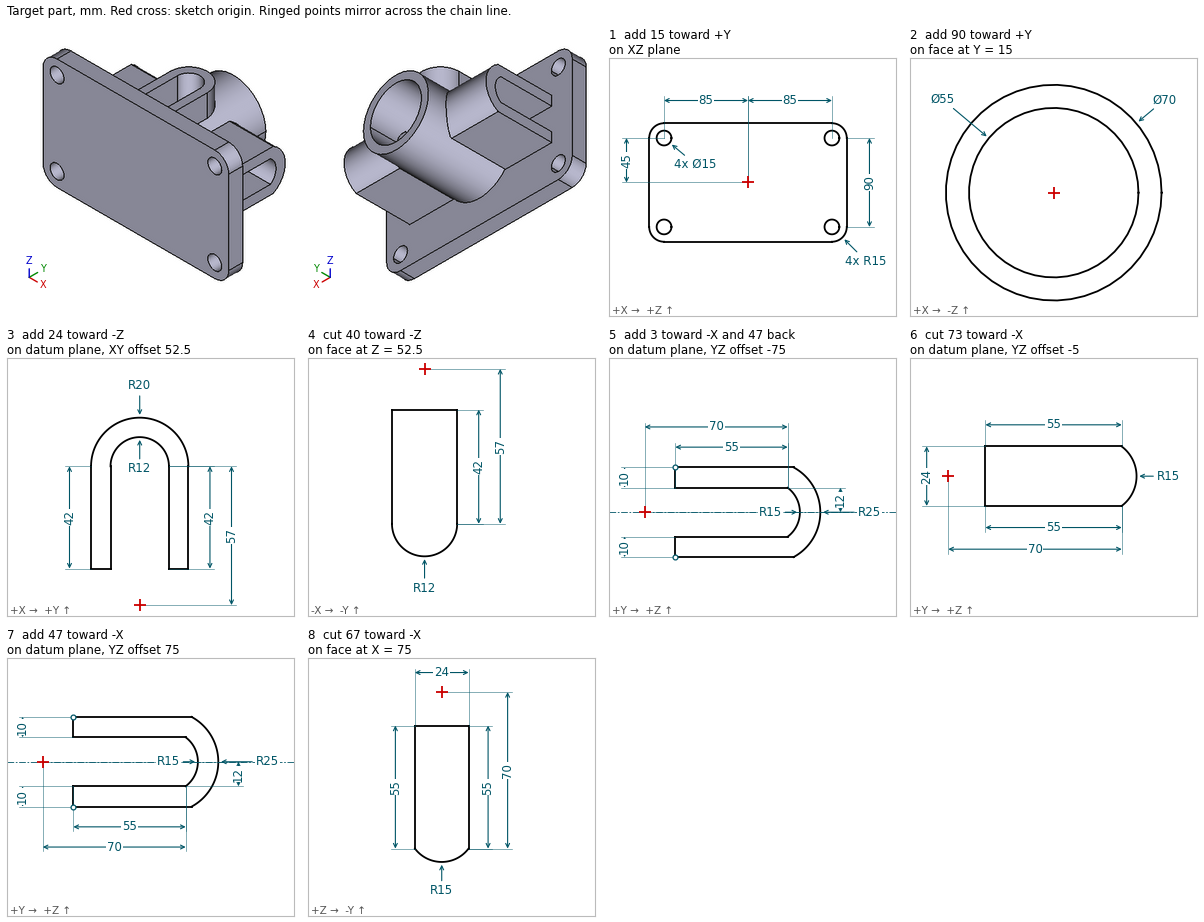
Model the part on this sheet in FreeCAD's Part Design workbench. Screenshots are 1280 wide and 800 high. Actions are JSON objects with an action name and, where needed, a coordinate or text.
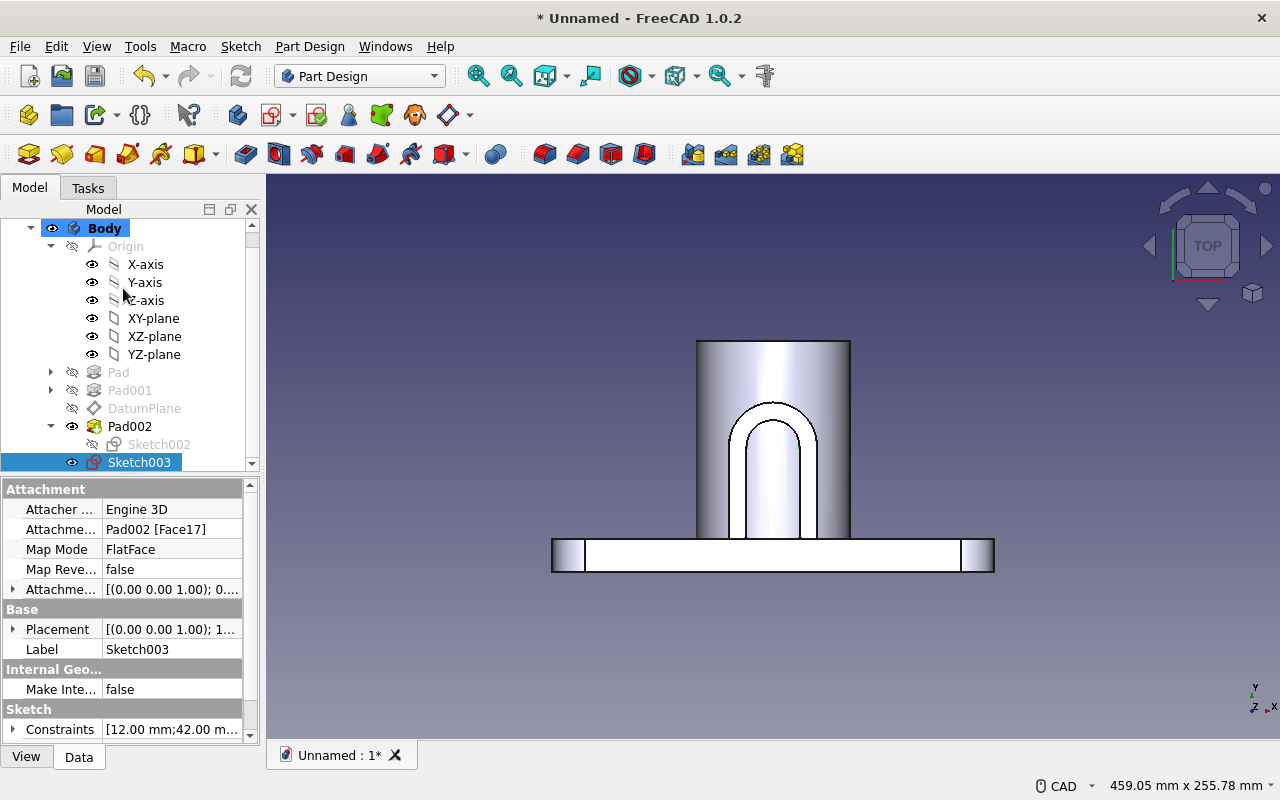
{"action": "left_click", "coordinate": [246, 154]}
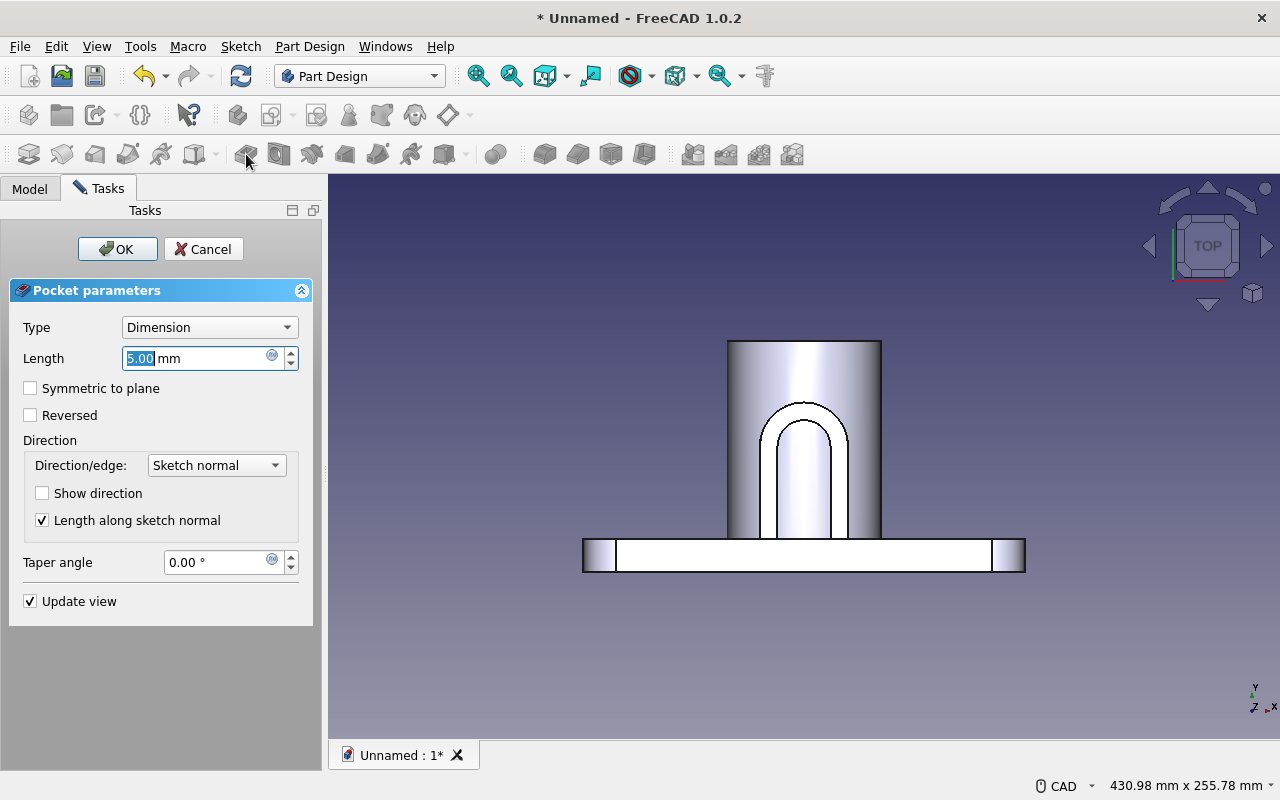
{"action": "type", "text": "40"}
{"action": "key", "text": "Tab"}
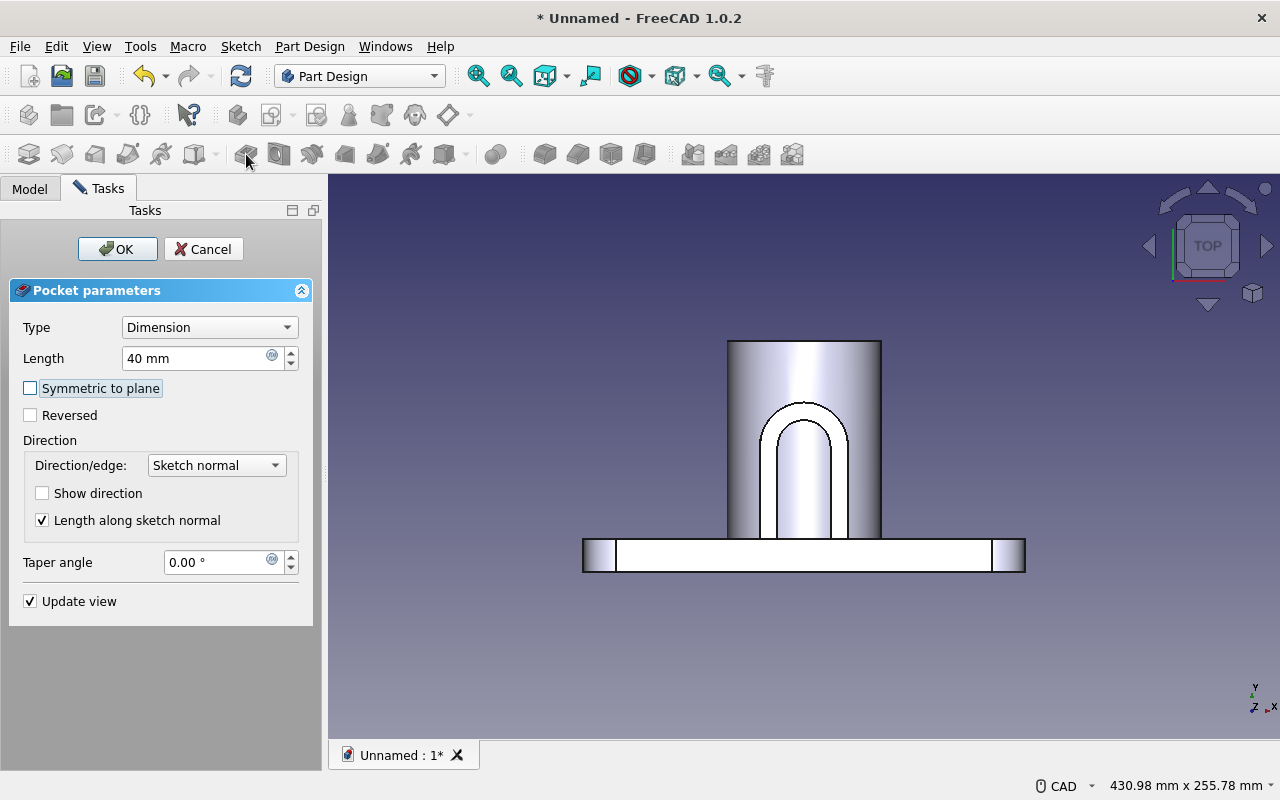
{"action": "left_click", "coordinate": [118, 249]}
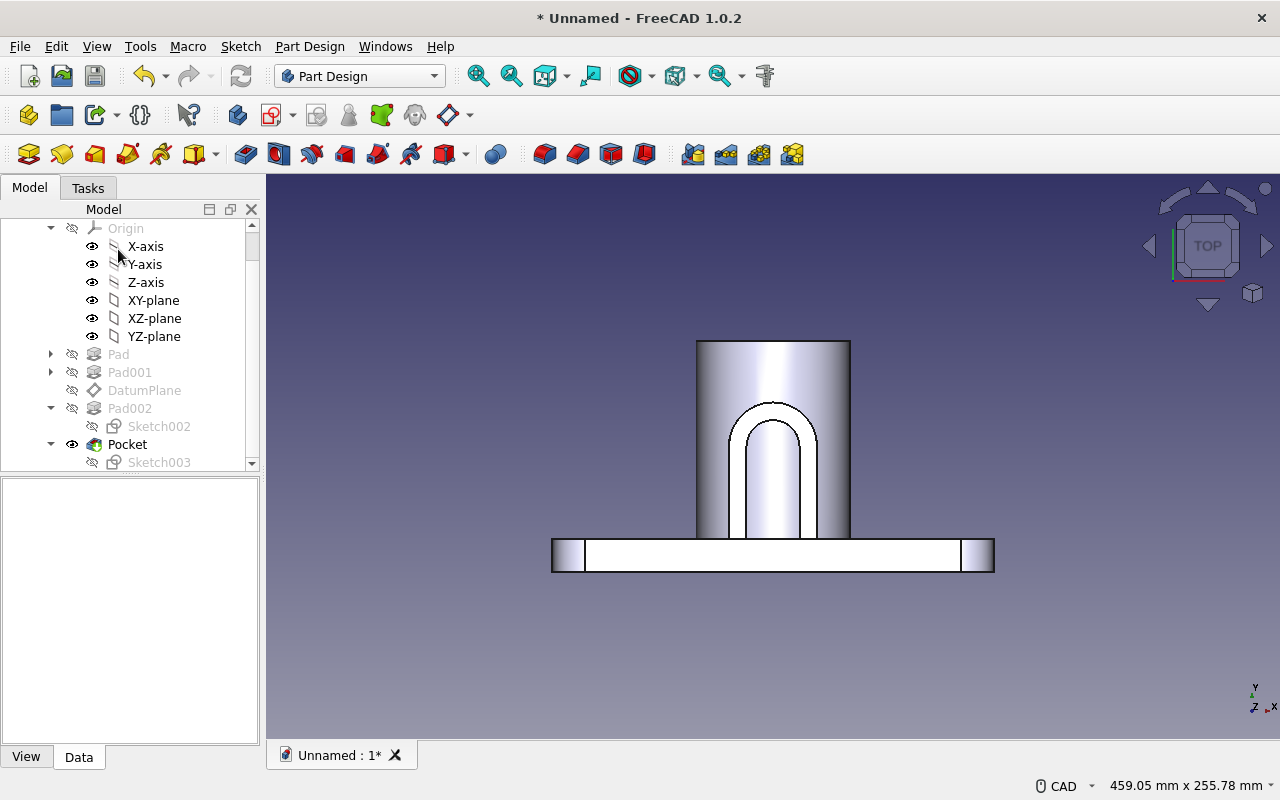
{"action": "left_click", "coordinate": [479, 76]}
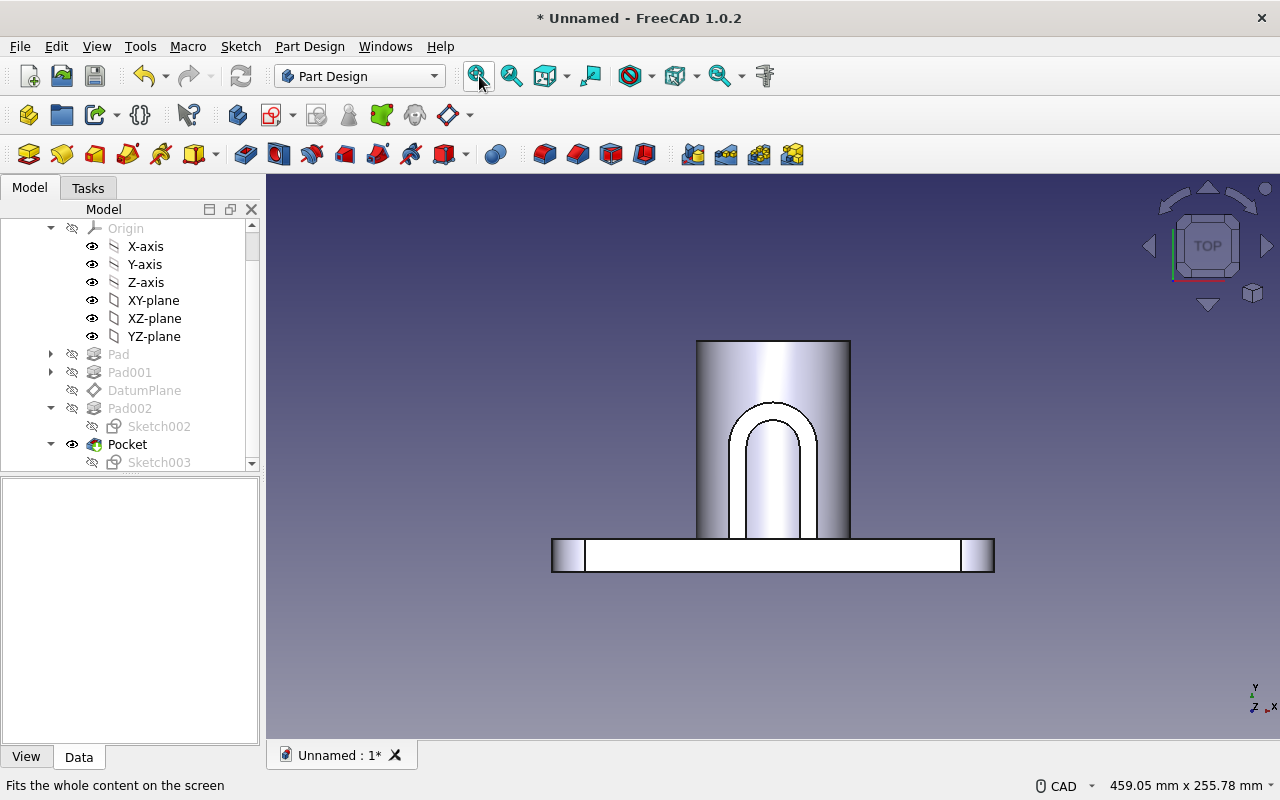
{"action": "left_click", "coordinate": [137, 336]}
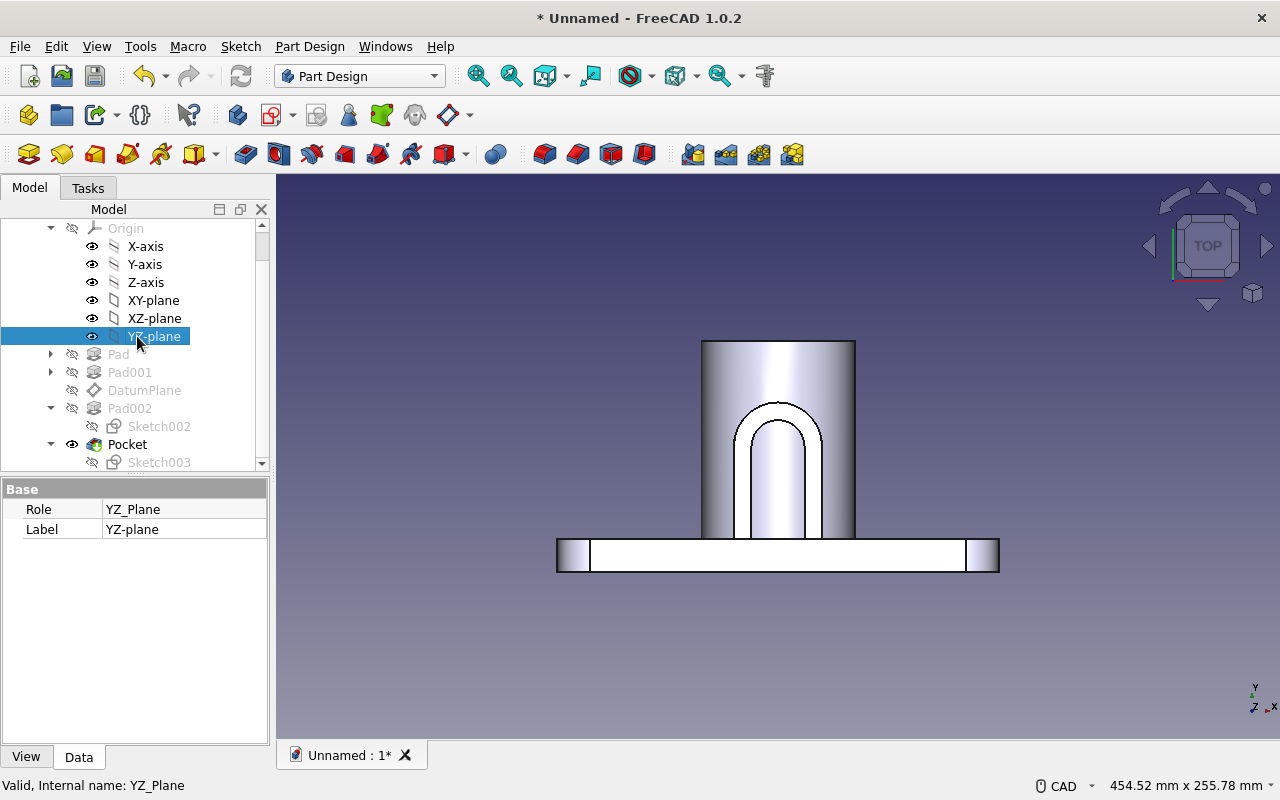
{"action": "left_click", "coordinate": [448, 116]}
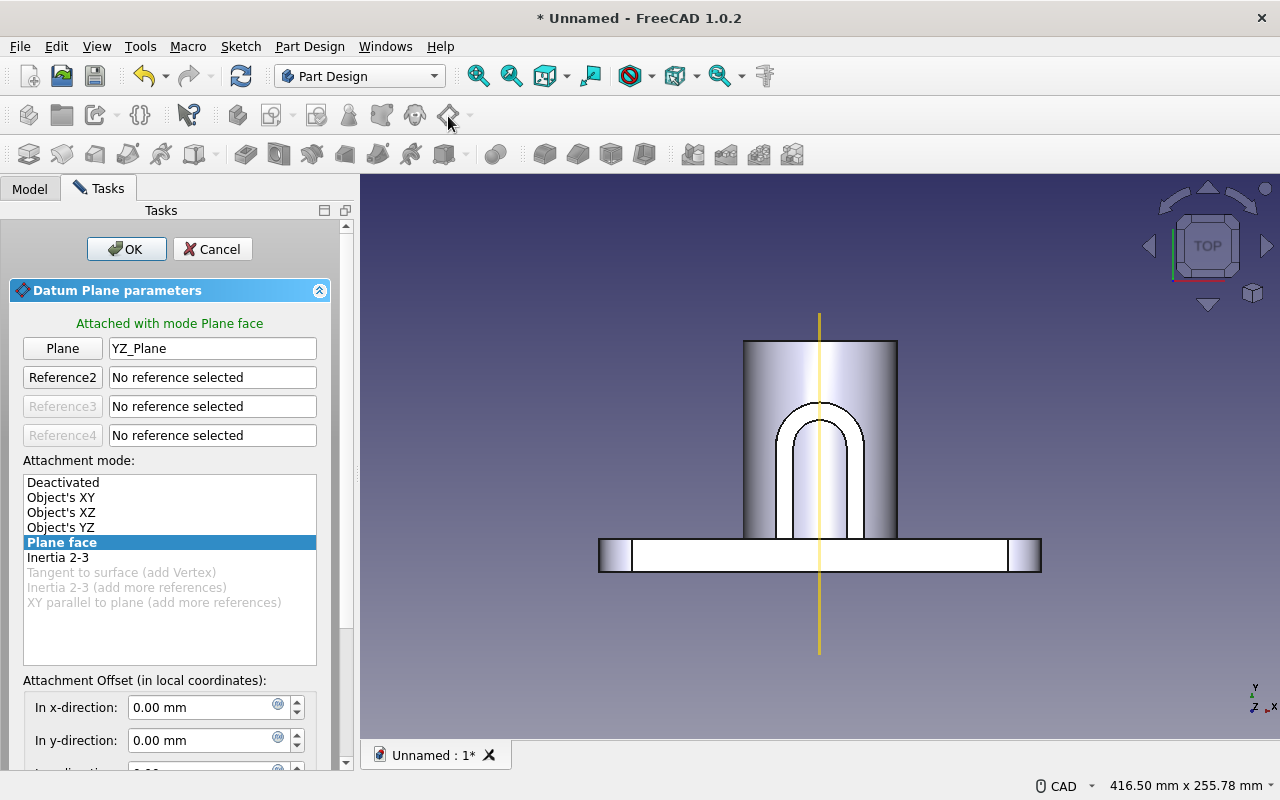
{"action": "scroll", "coordinate": [346, 495], "scroll_direction": "down", "scroll_amount": 2}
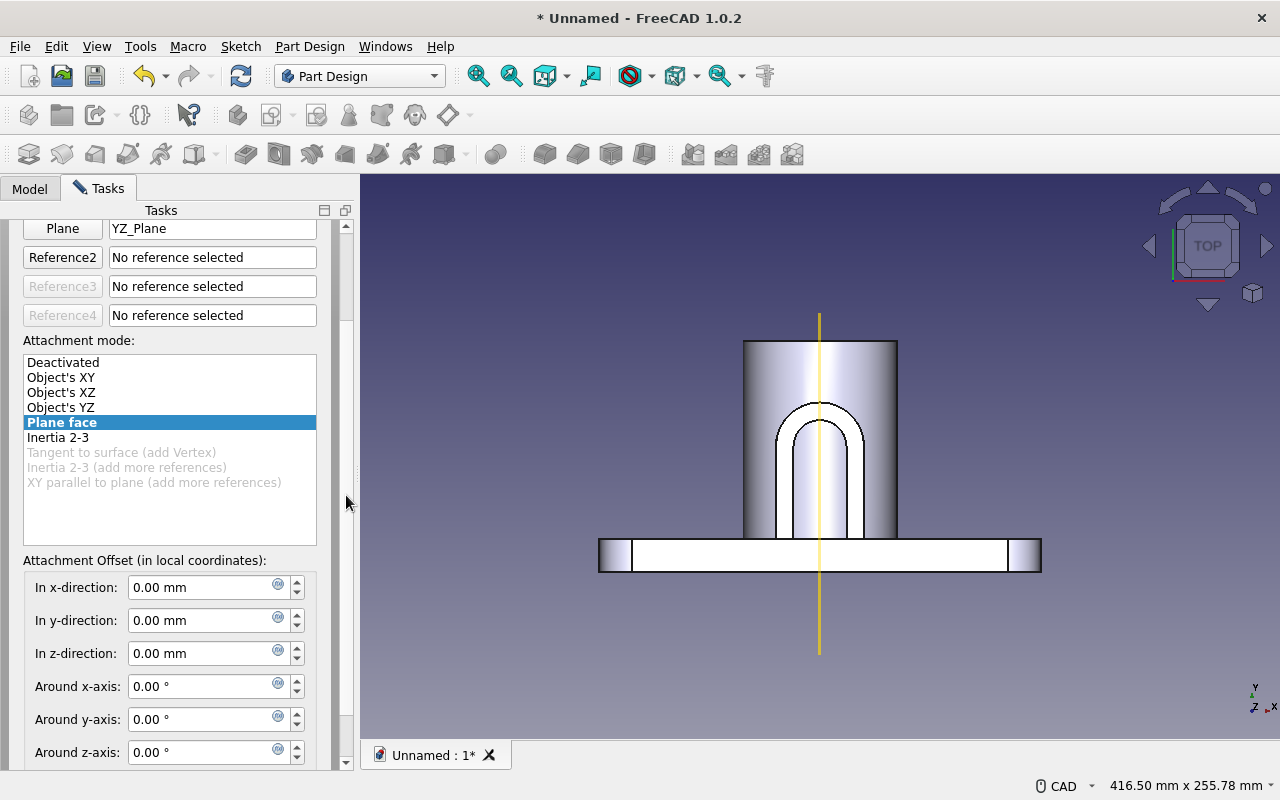
{"action": "triple_click", "coordinate": [210, 654]}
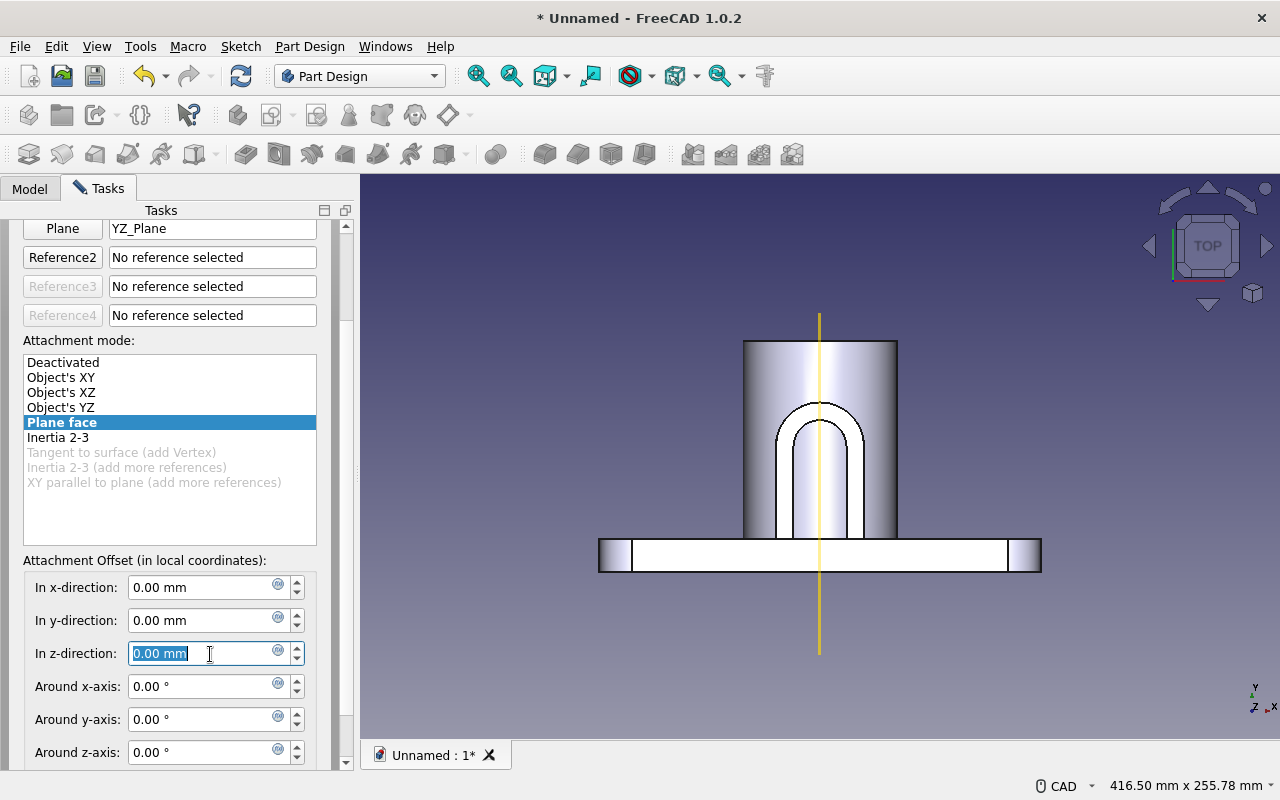
{"action": "type", "text": "-75"}
{"action": "key", "text": "Tab"}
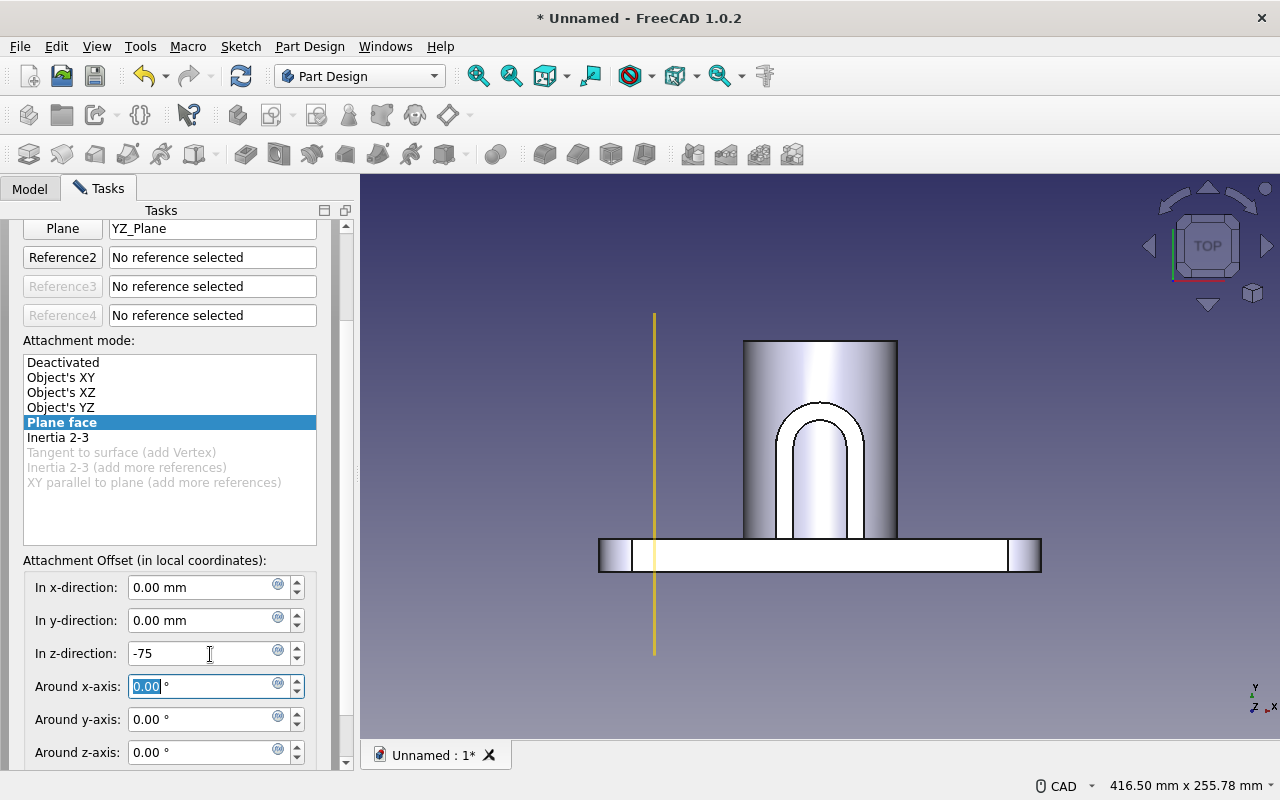
{"action": "scroll", "coordinate": [346, 495], "scroll_direction": "up", "scroll_amount": 3}